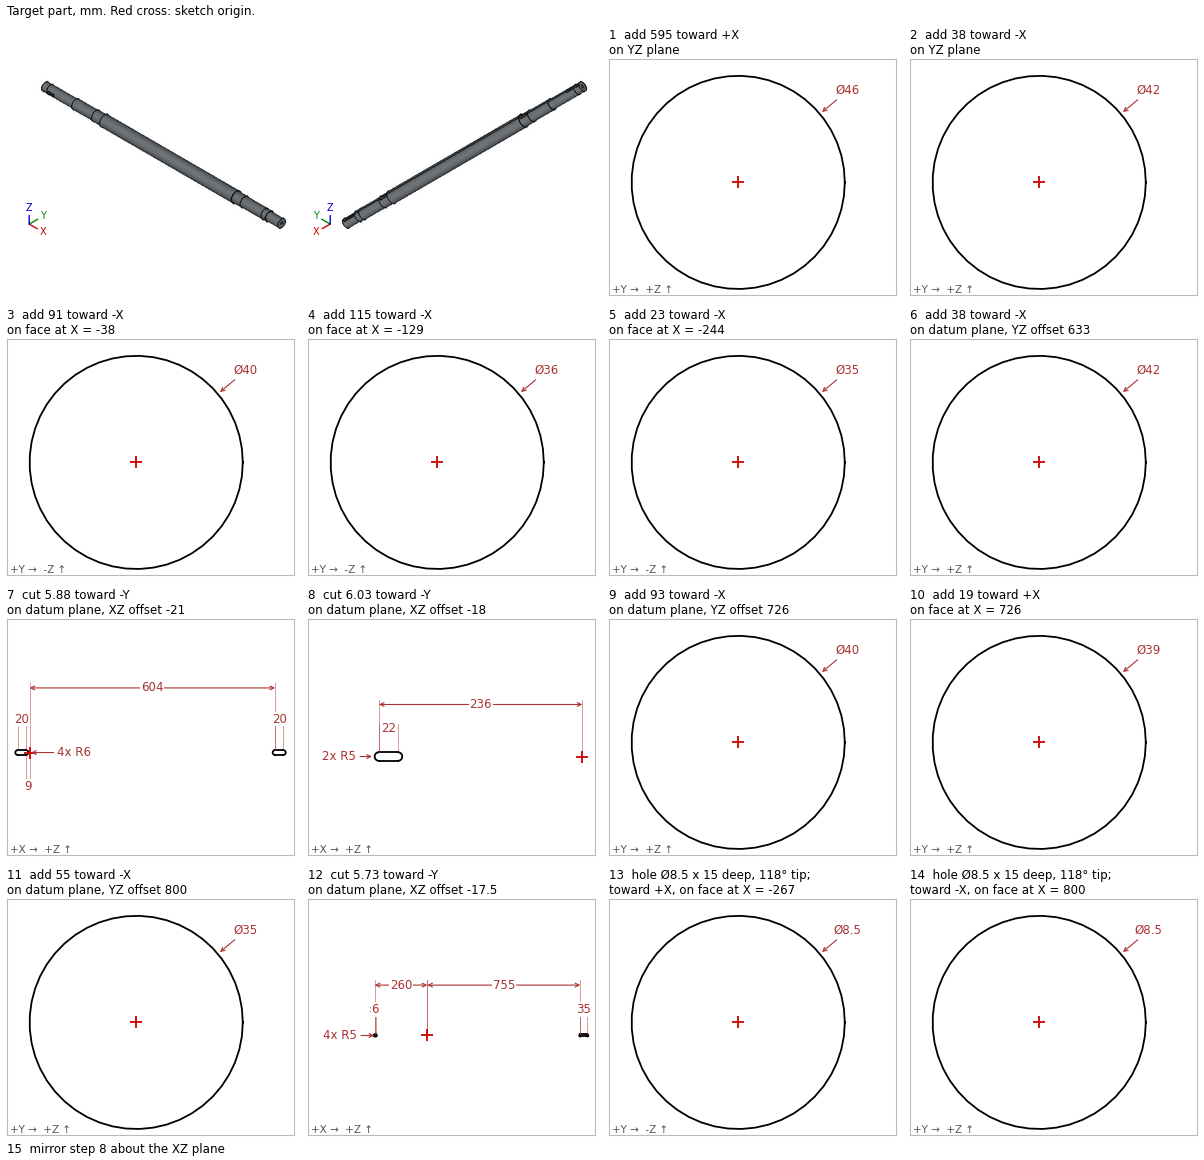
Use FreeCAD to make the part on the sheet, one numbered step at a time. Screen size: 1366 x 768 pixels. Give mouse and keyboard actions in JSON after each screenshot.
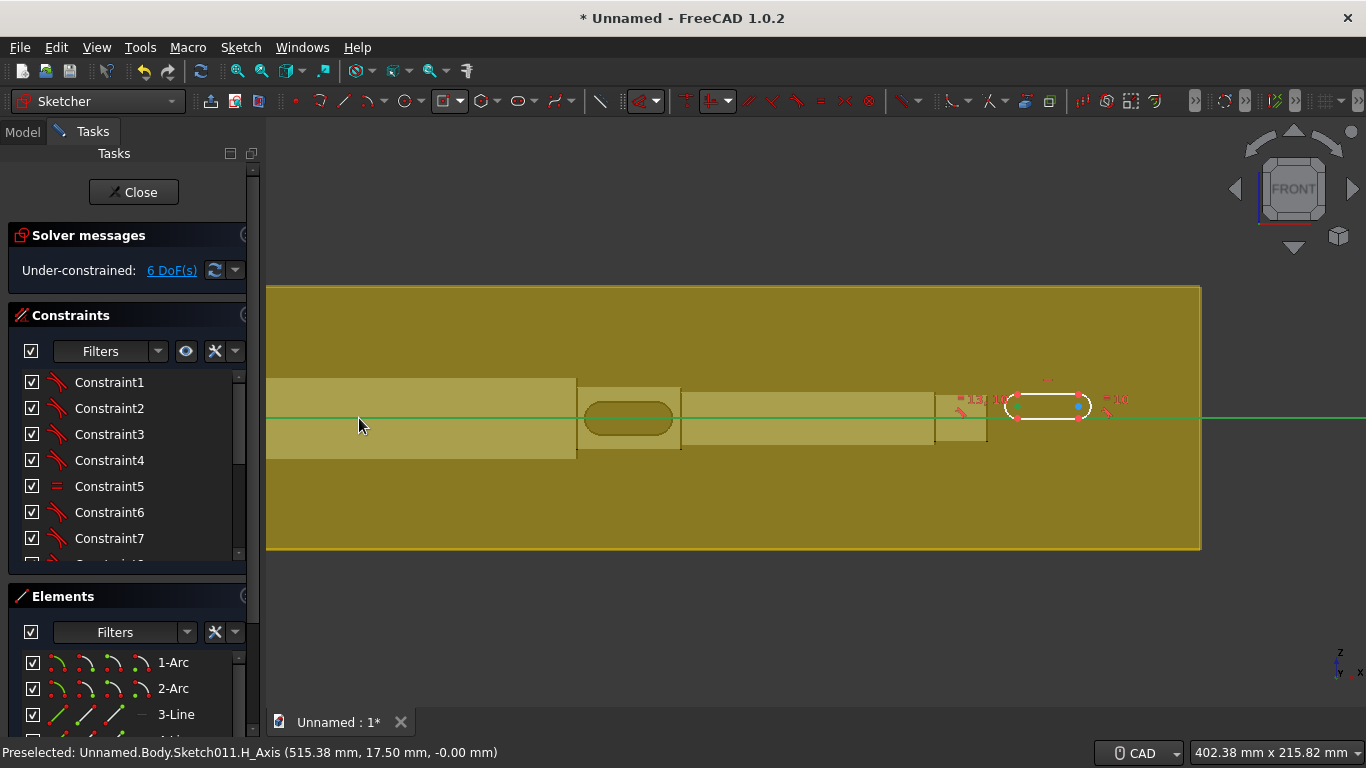
{"action": "key", "text": "c"}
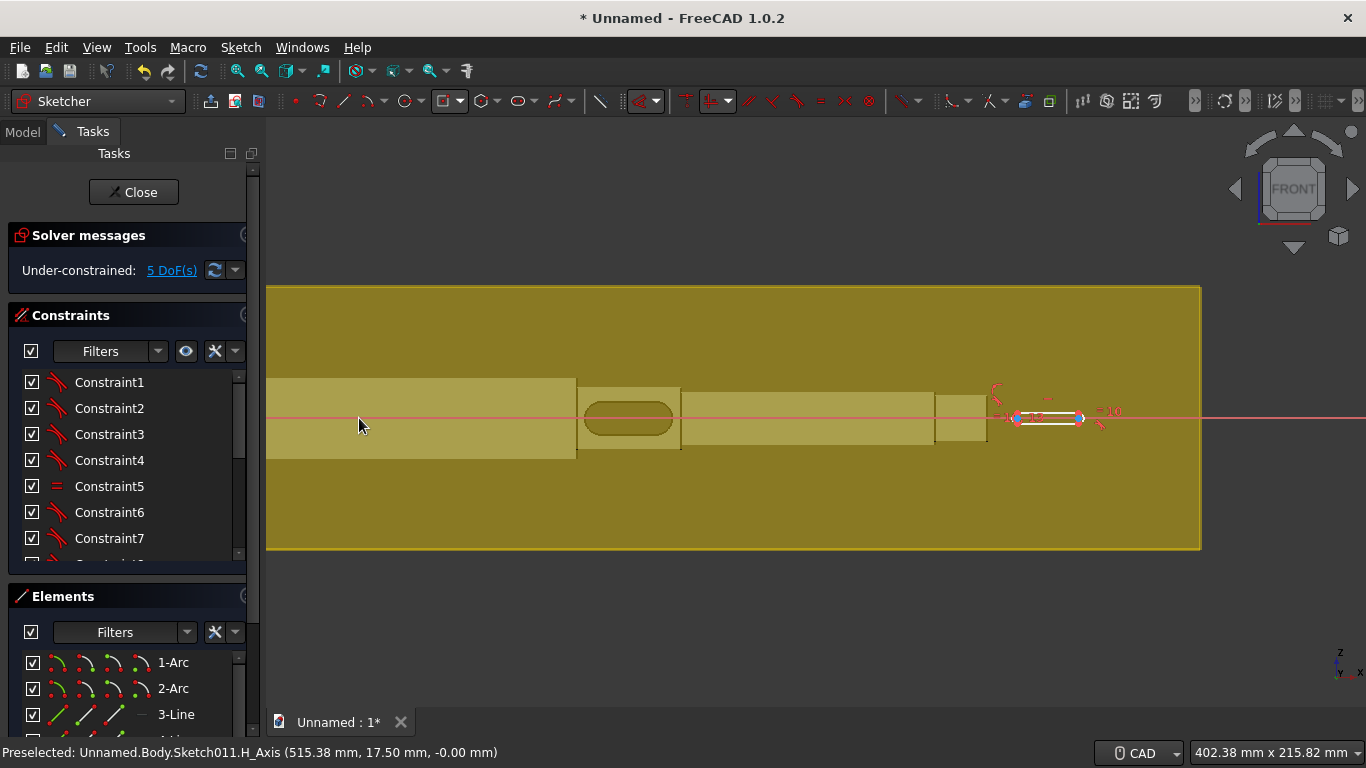
{"action": "scroll", "coordinate": [1019, 410], "scroll_direction": "down", "scroll_amount": 8}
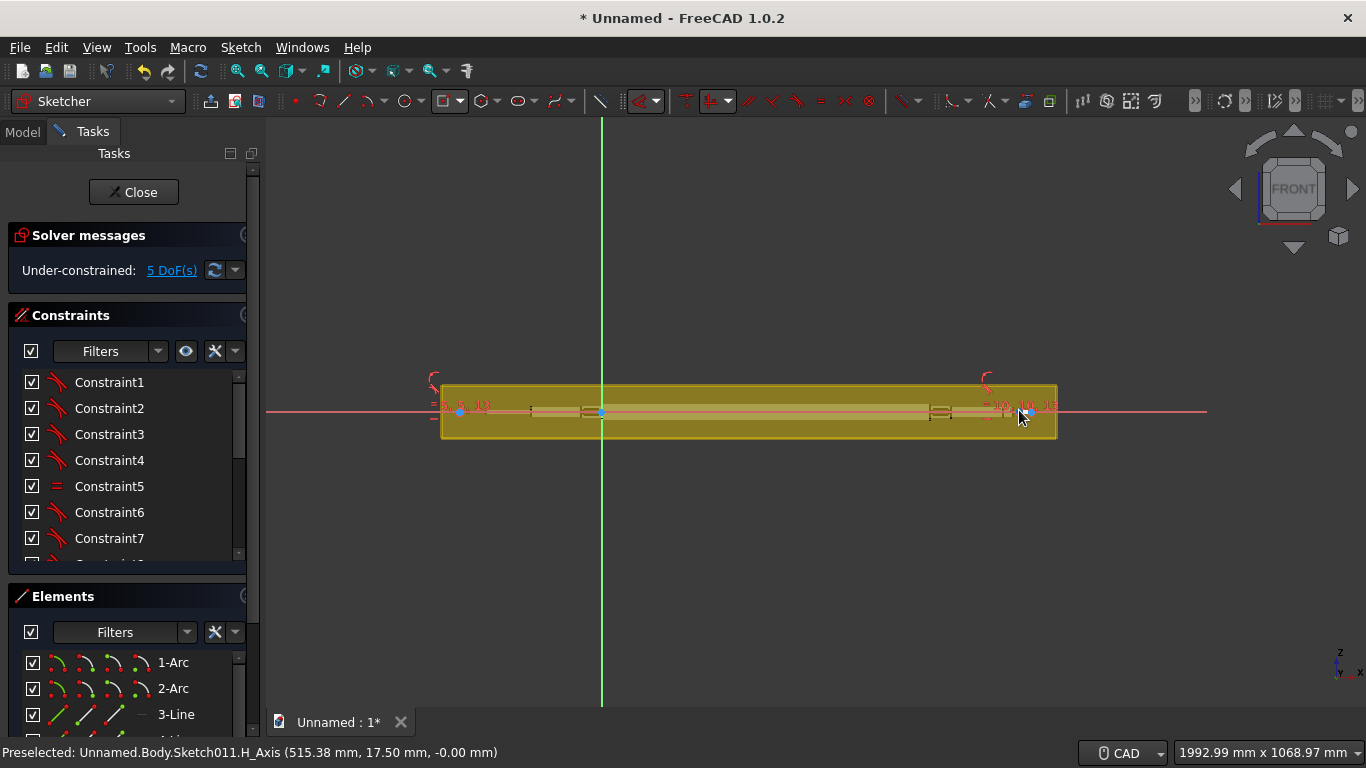
{"action": "scroll", "coordinate": [459, 412], "scroll_direction": "up", "scroll_amount": 14}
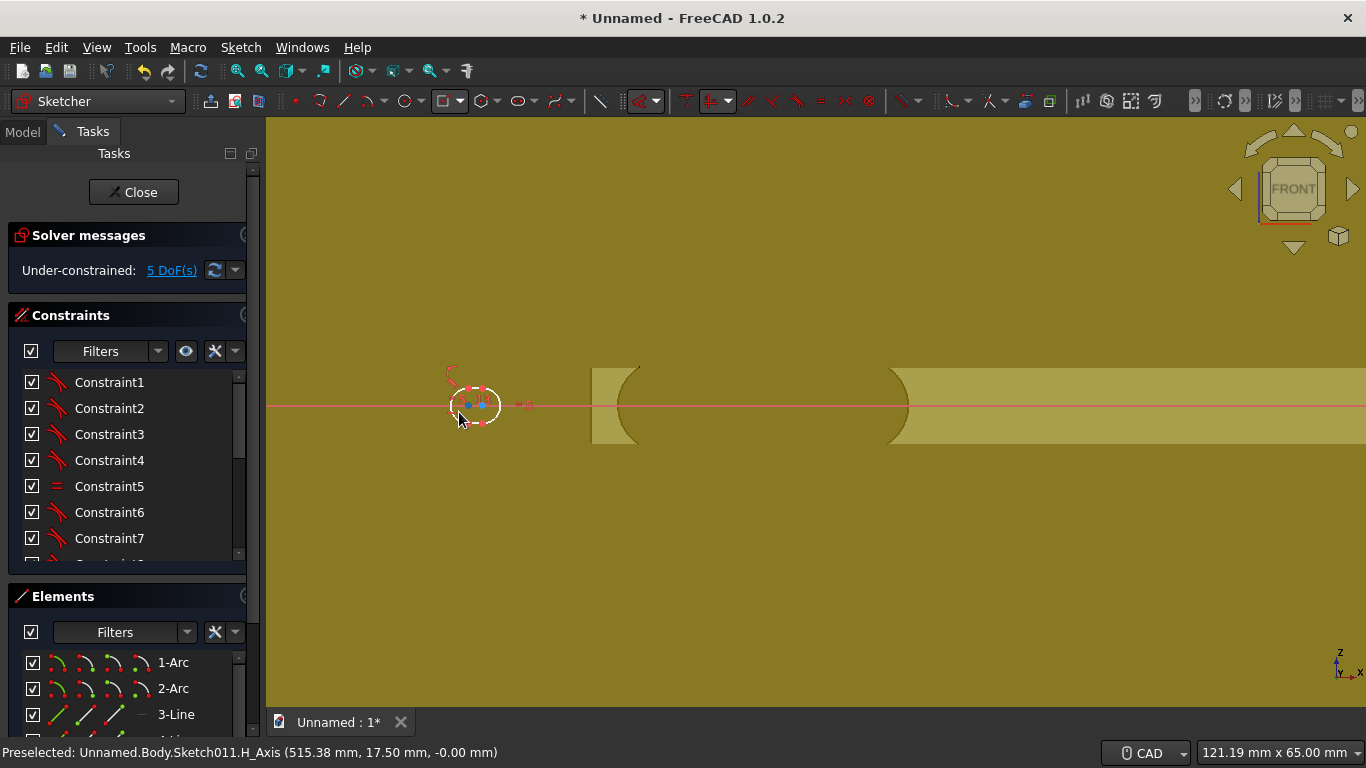
{"action": "left_click", "coordinate": [458, 420]}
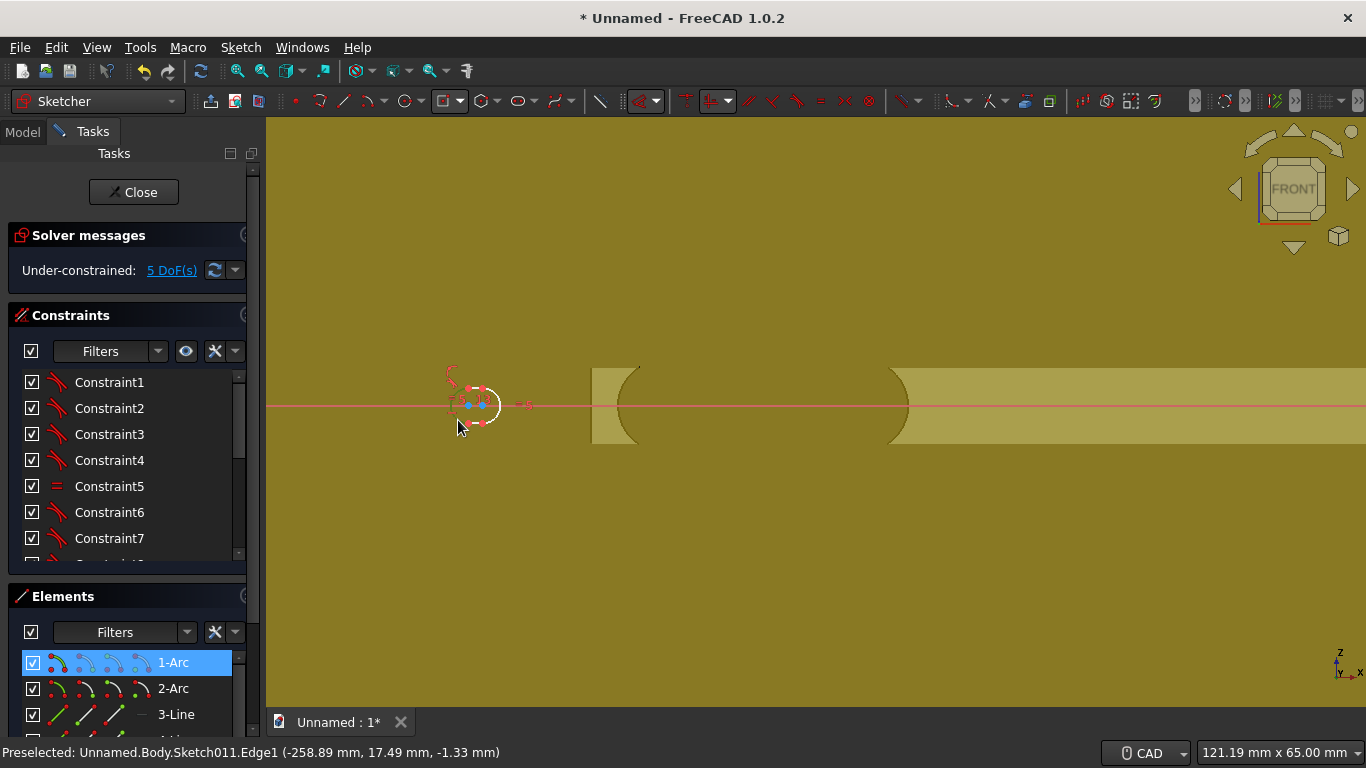
{"action": "left_click", "coordinate": [658, 102]}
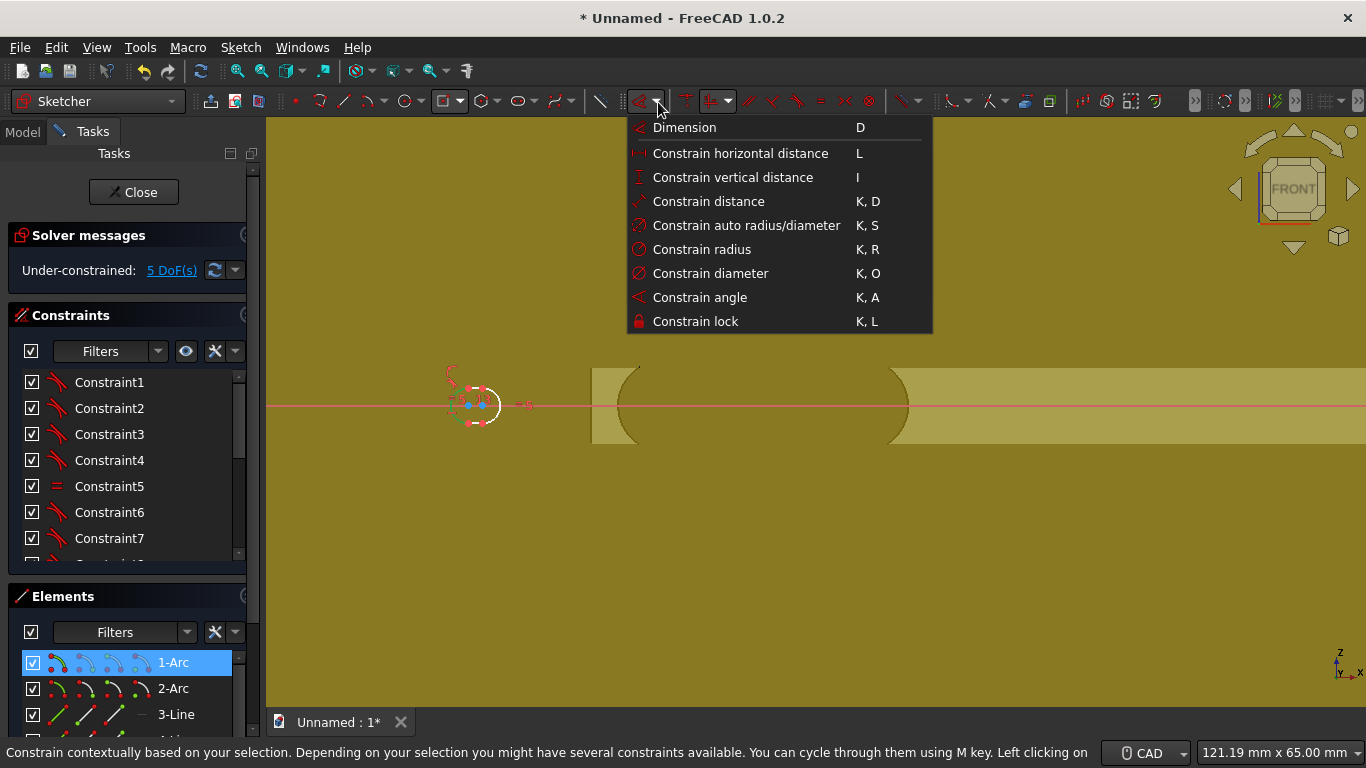
{"action": "left_click", "coordinate": [780, 249]}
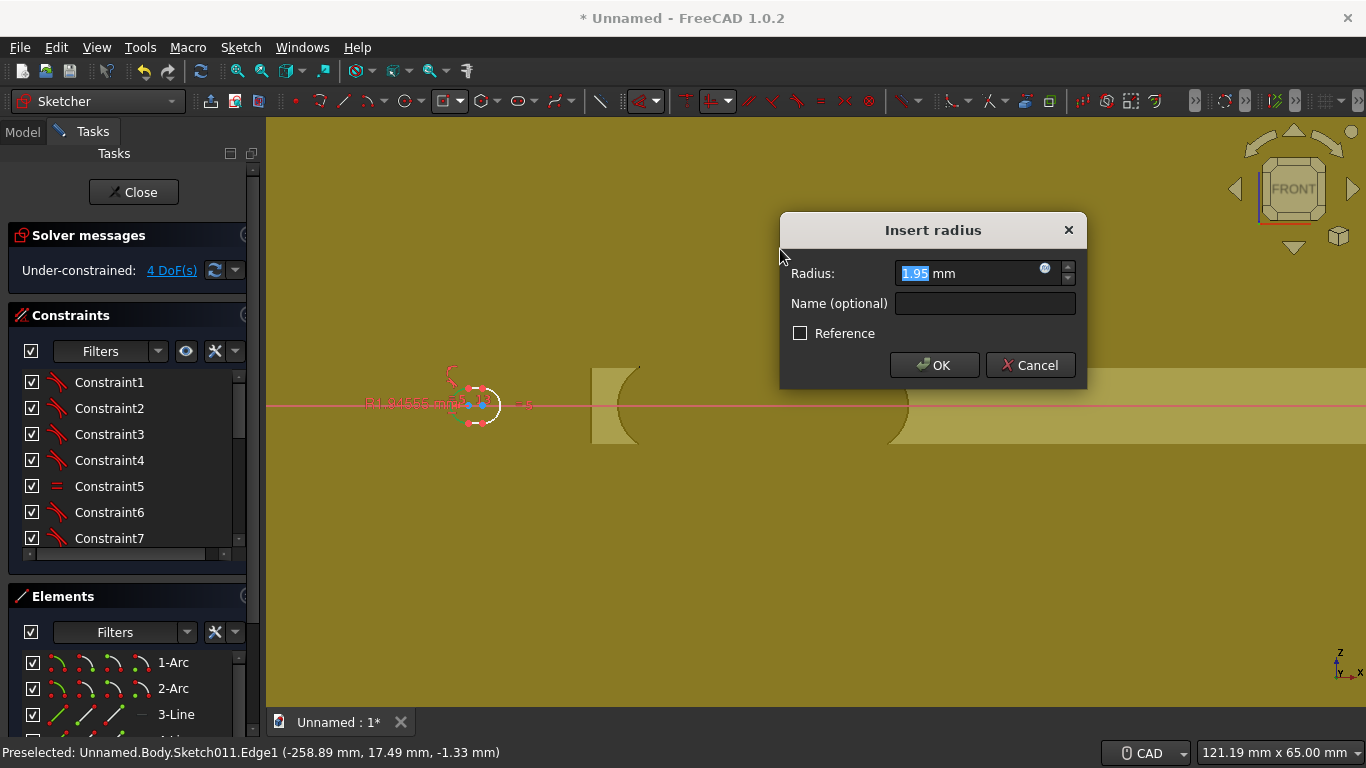
{"action": "type", "text": "5"}
{"action": "key", "text": "Return"}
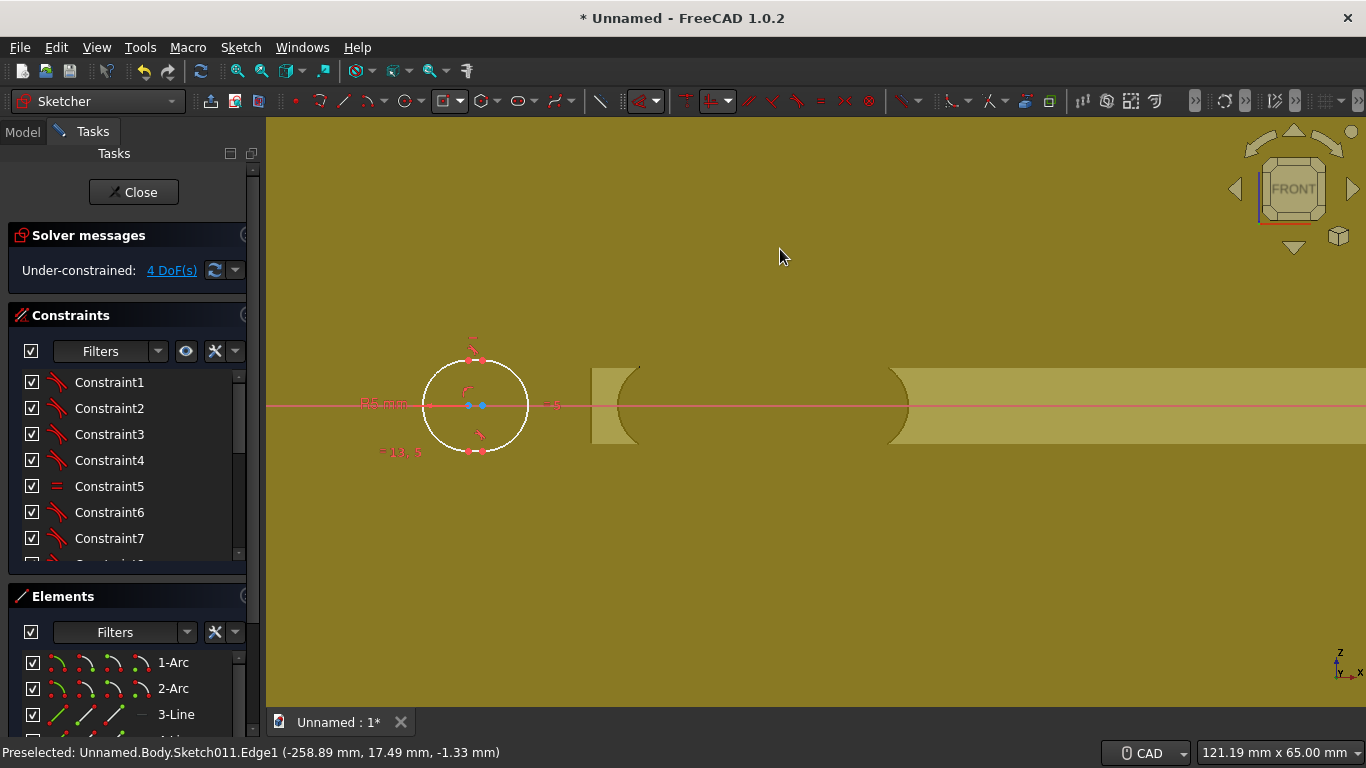
{"action": "left_click", "coordinate": [475, 360]}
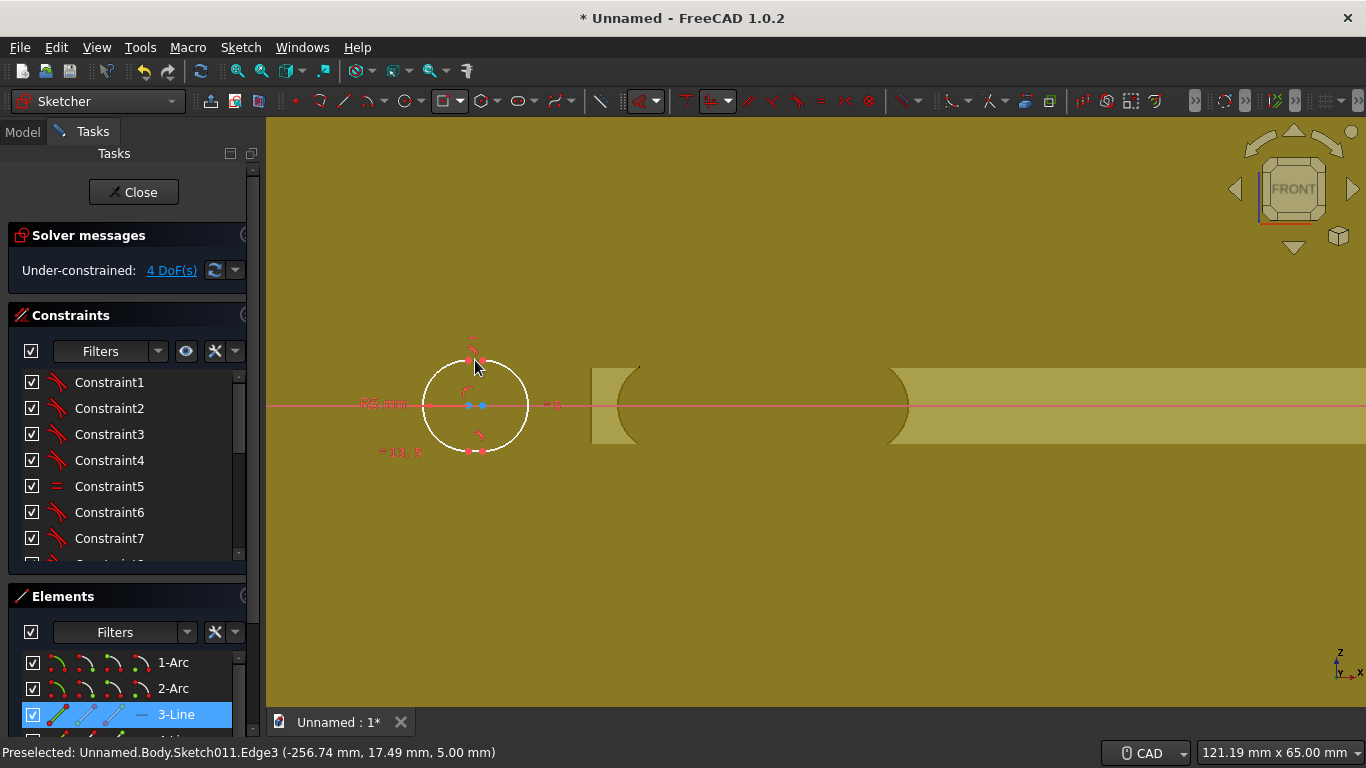
{"action": "key", "text": "l"}